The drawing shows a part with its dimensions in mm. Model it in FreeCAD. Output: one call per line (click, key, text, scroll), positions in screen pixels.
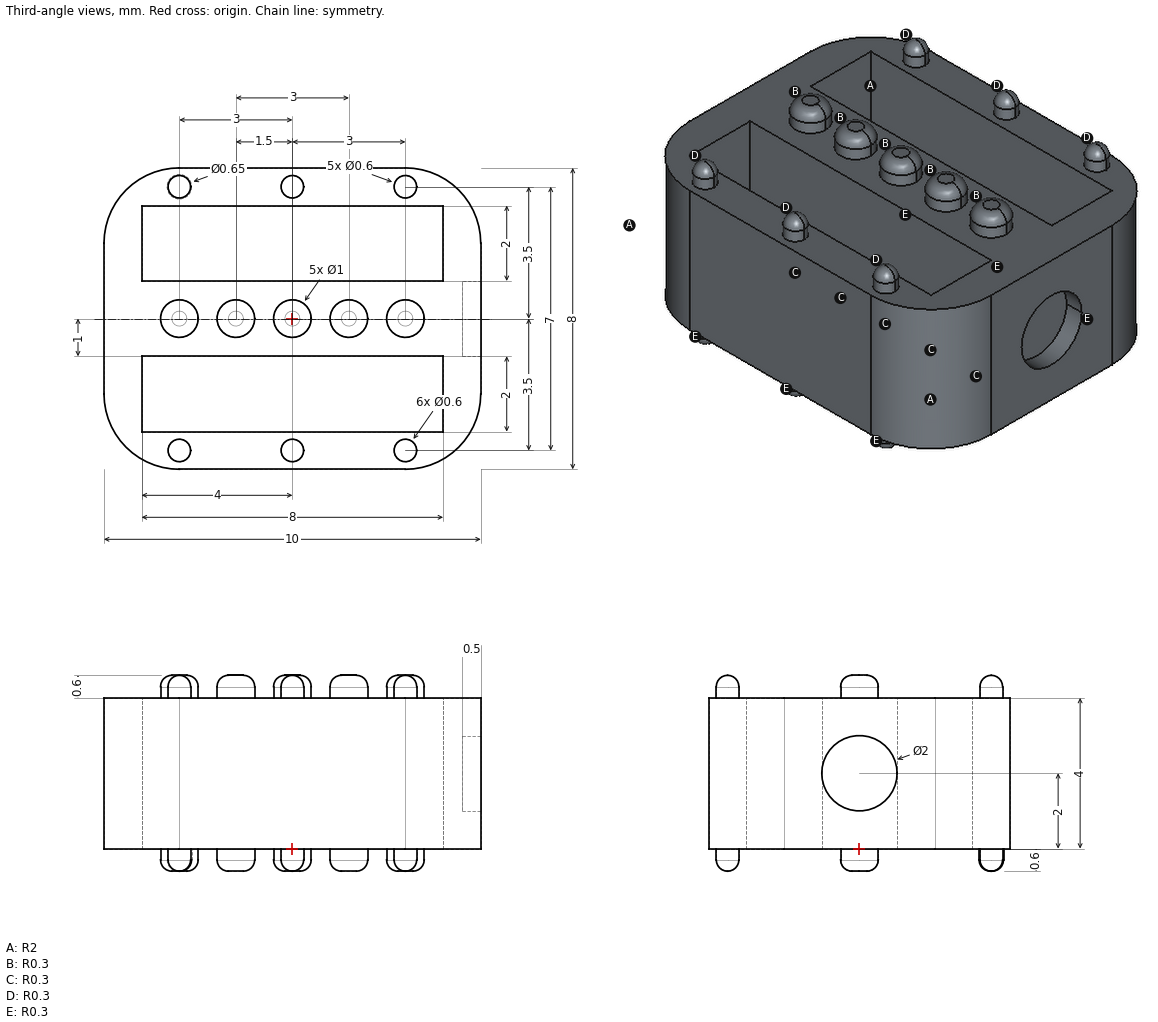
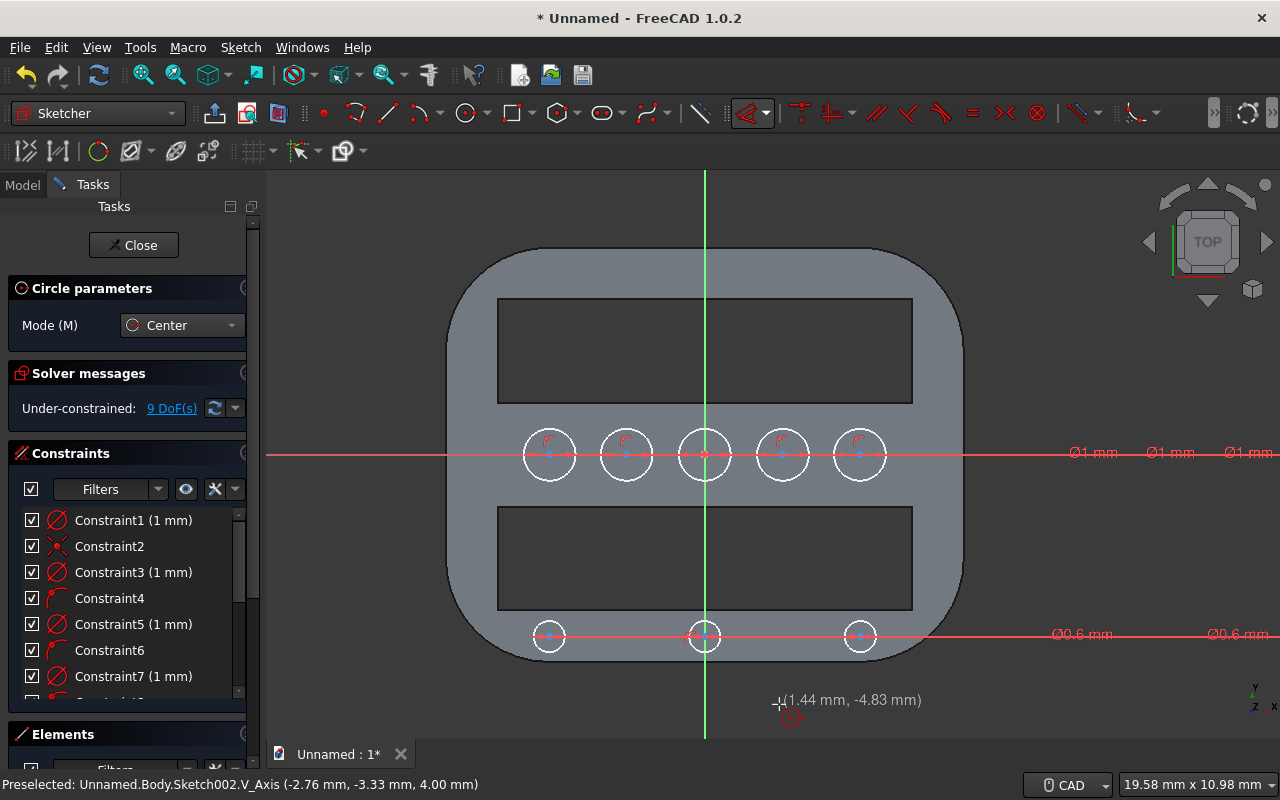
scroll(860, 274, up, 2)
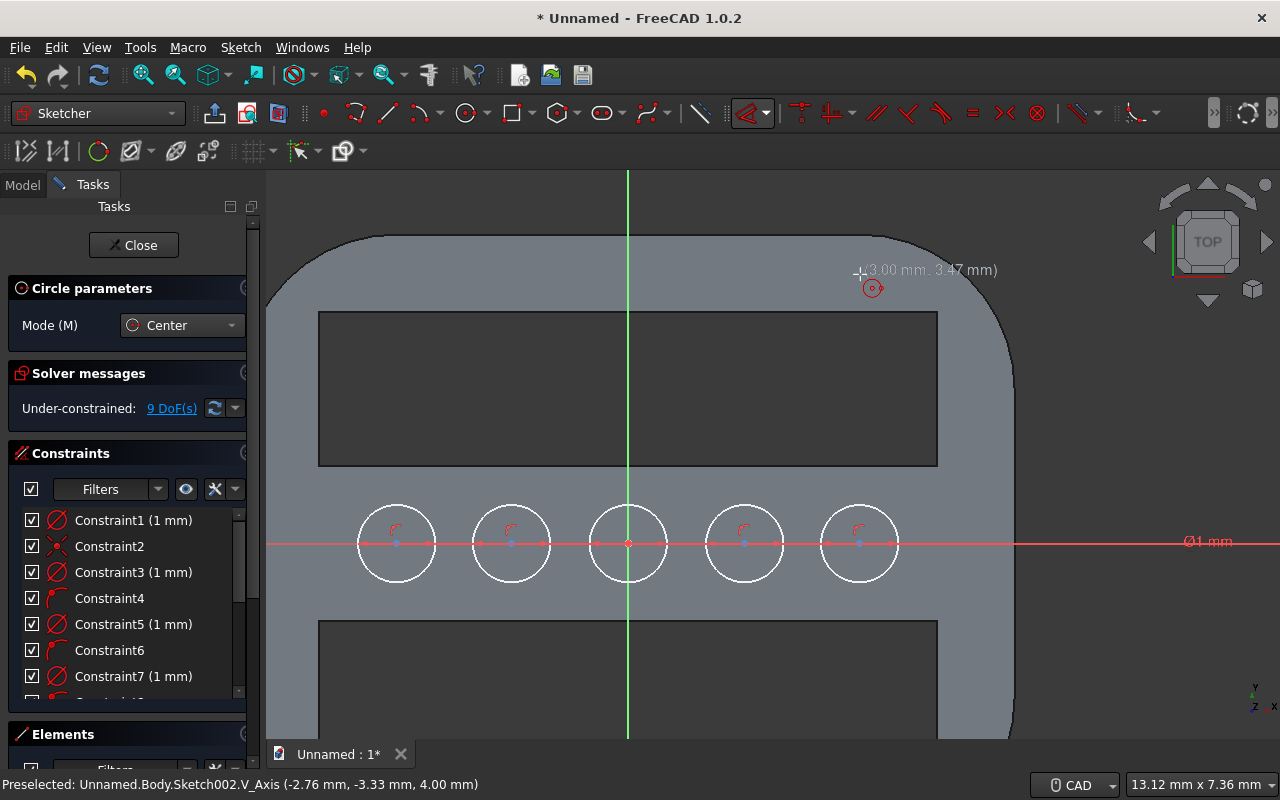
click(860, 273)
move(876, 257)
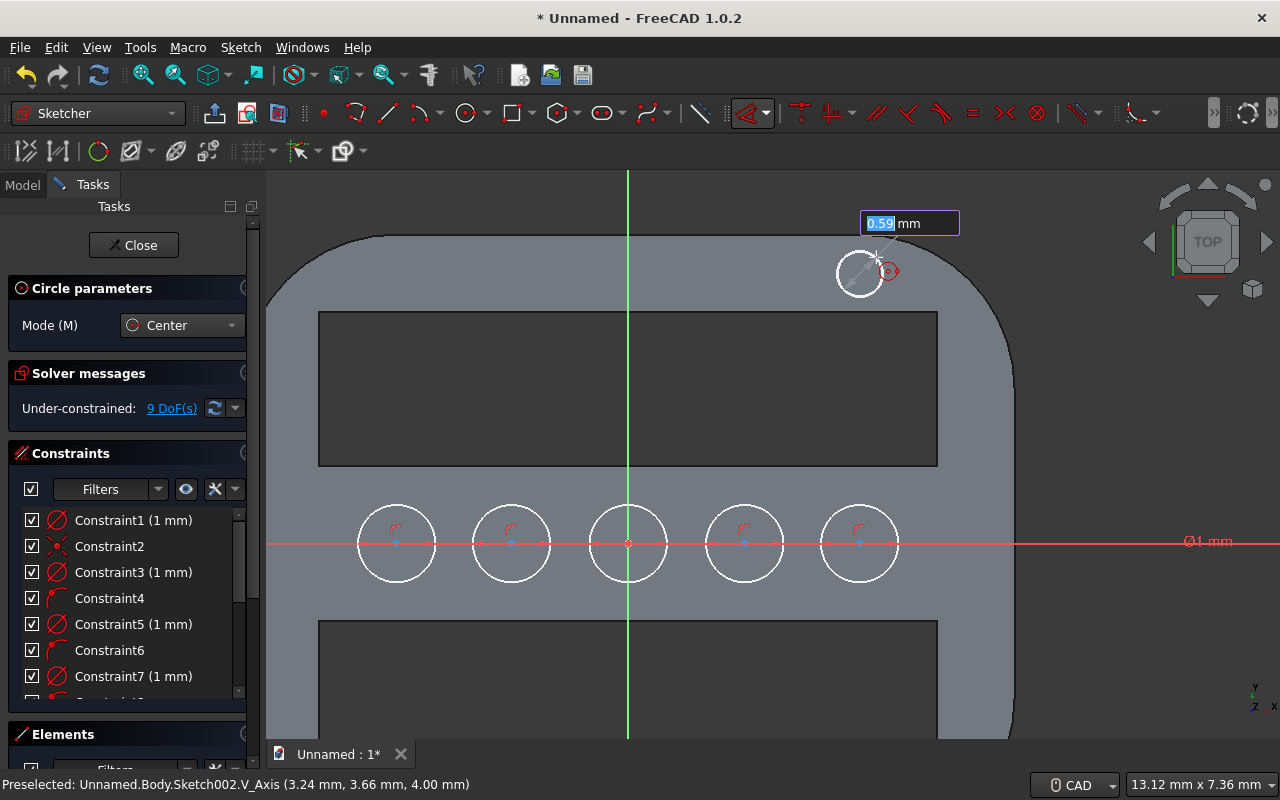
text(0.6)
key(Return)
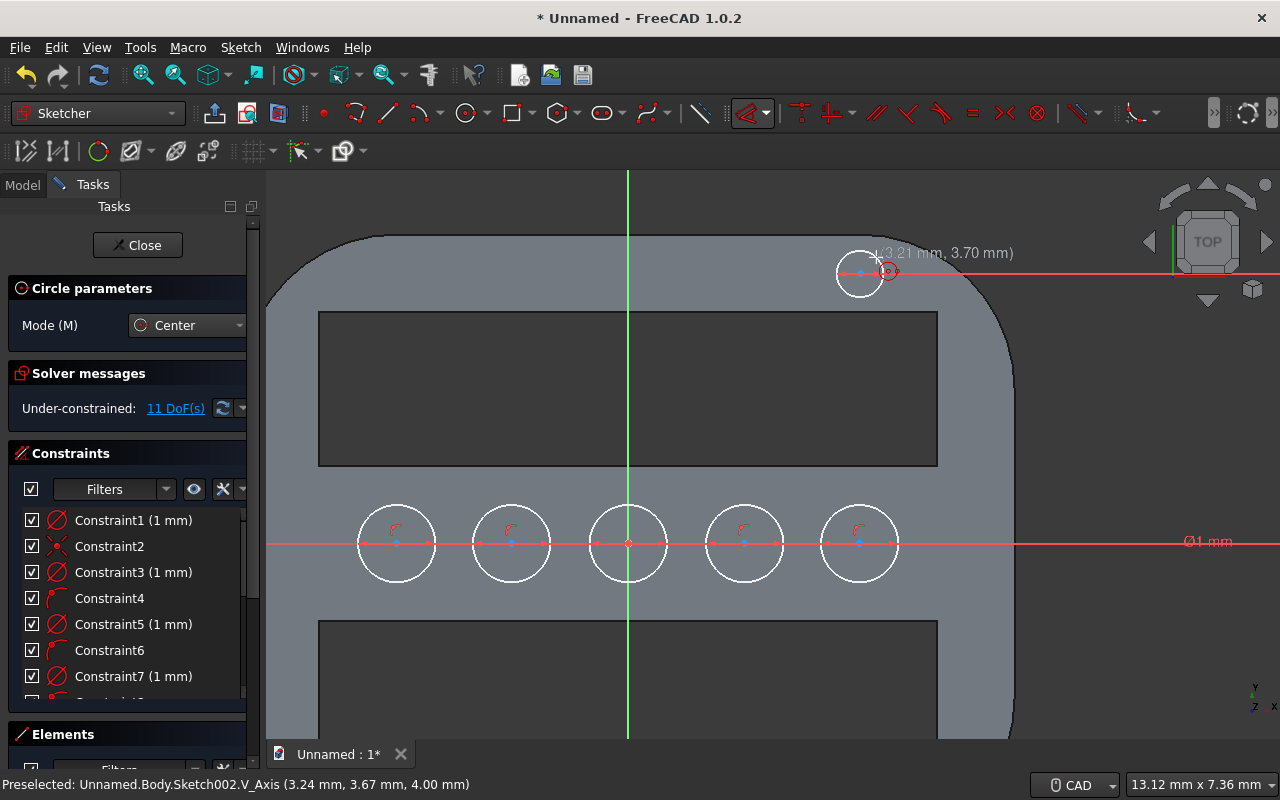
click(628, 273)
move(645, 257)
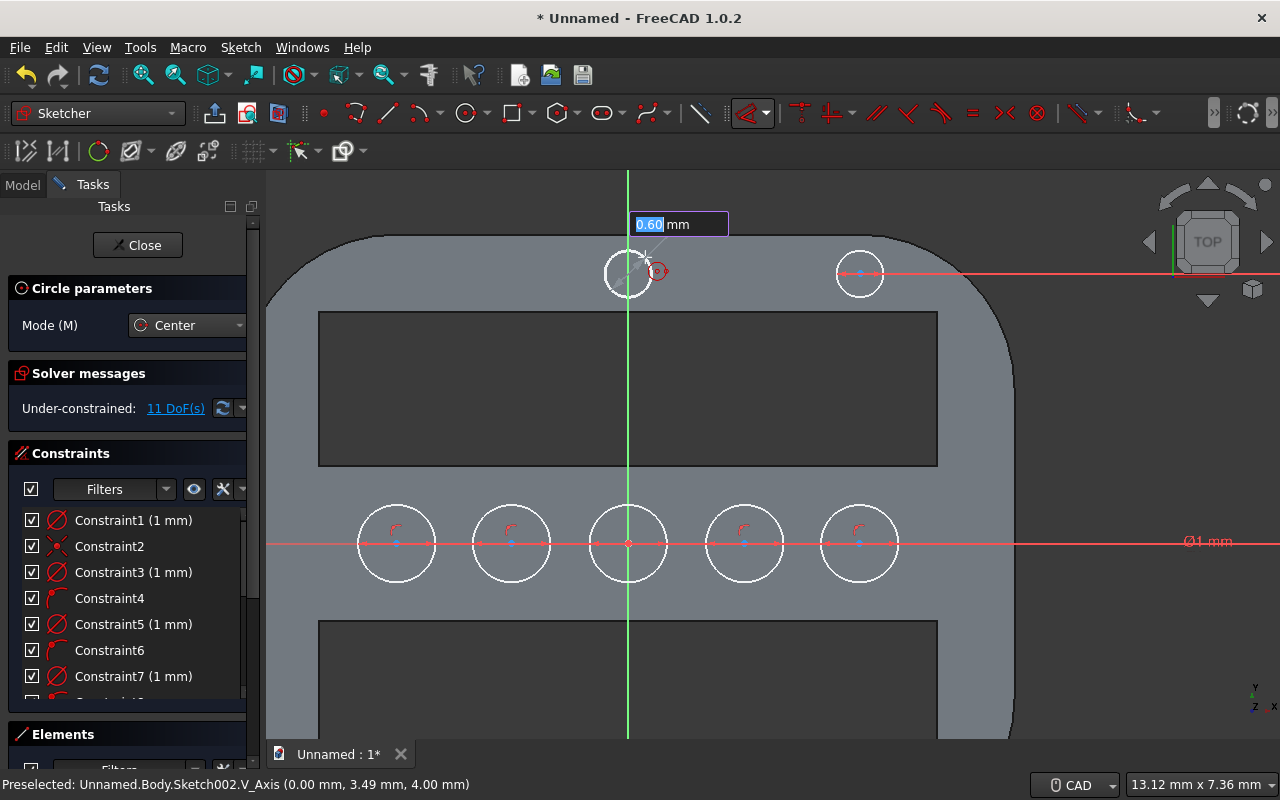
text(0.6)
key(Return)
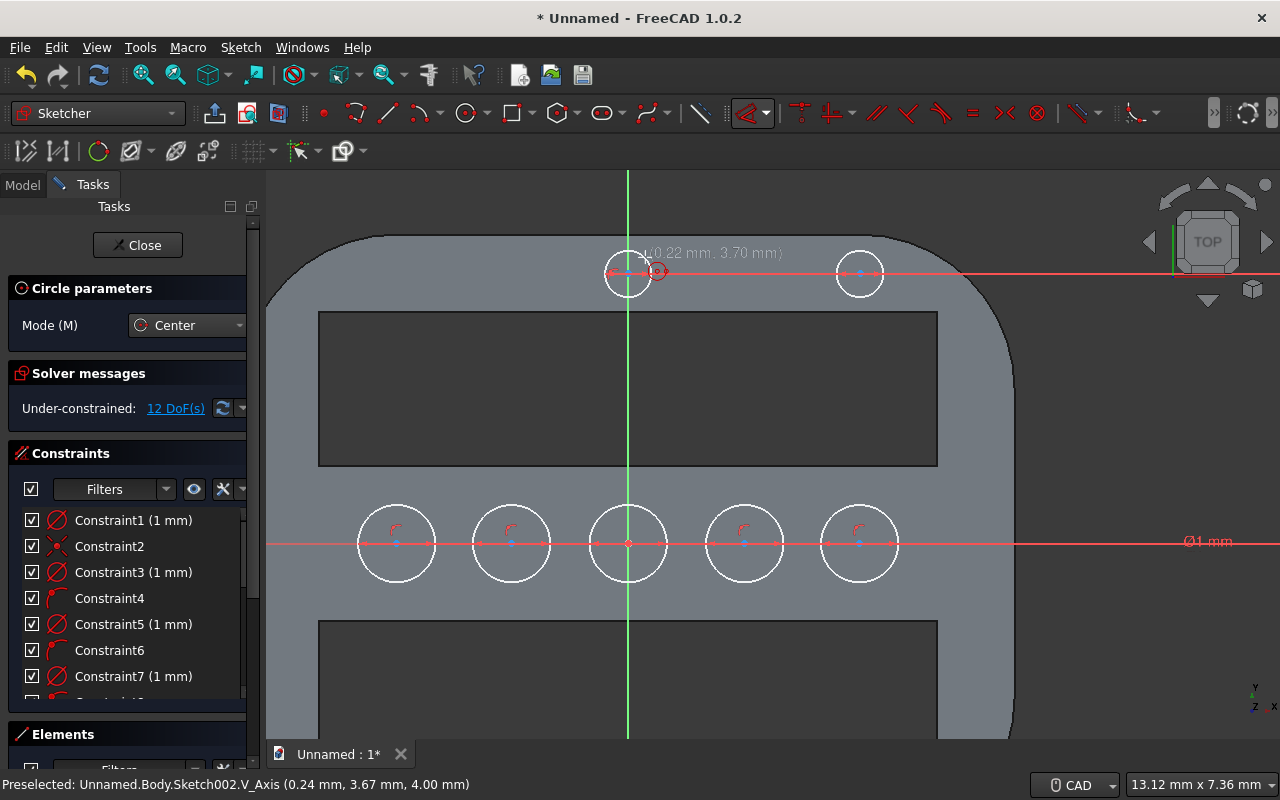
click(396, 273)
move(413, 257)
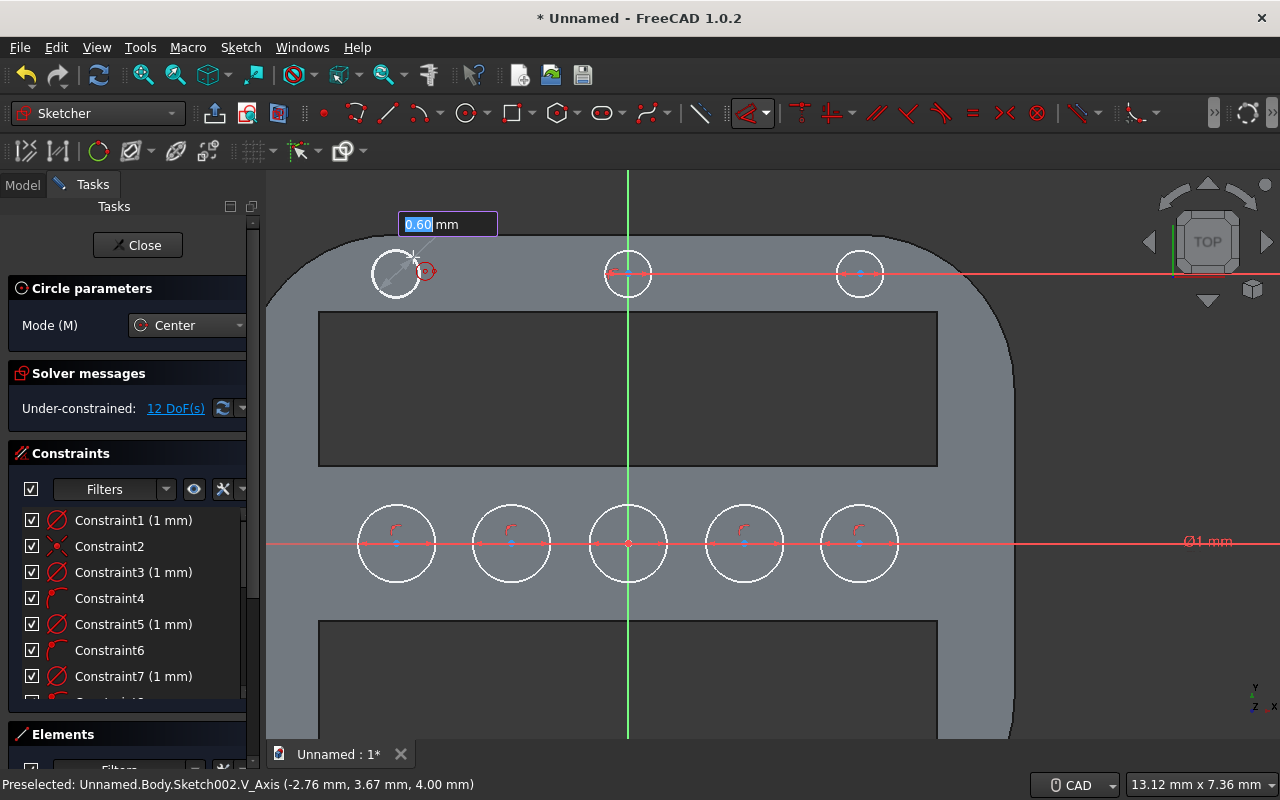
text(0.6)
key(Return)
key(Escape)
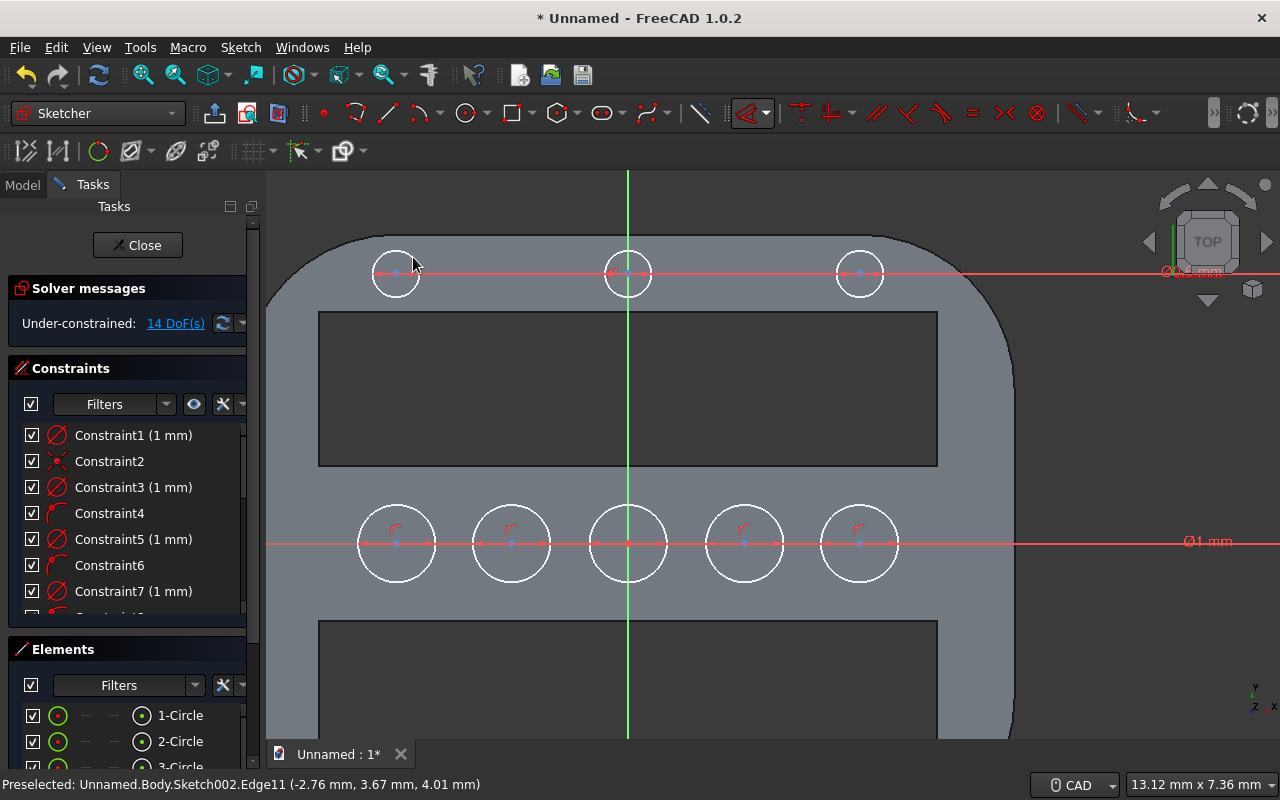
click(860, 544)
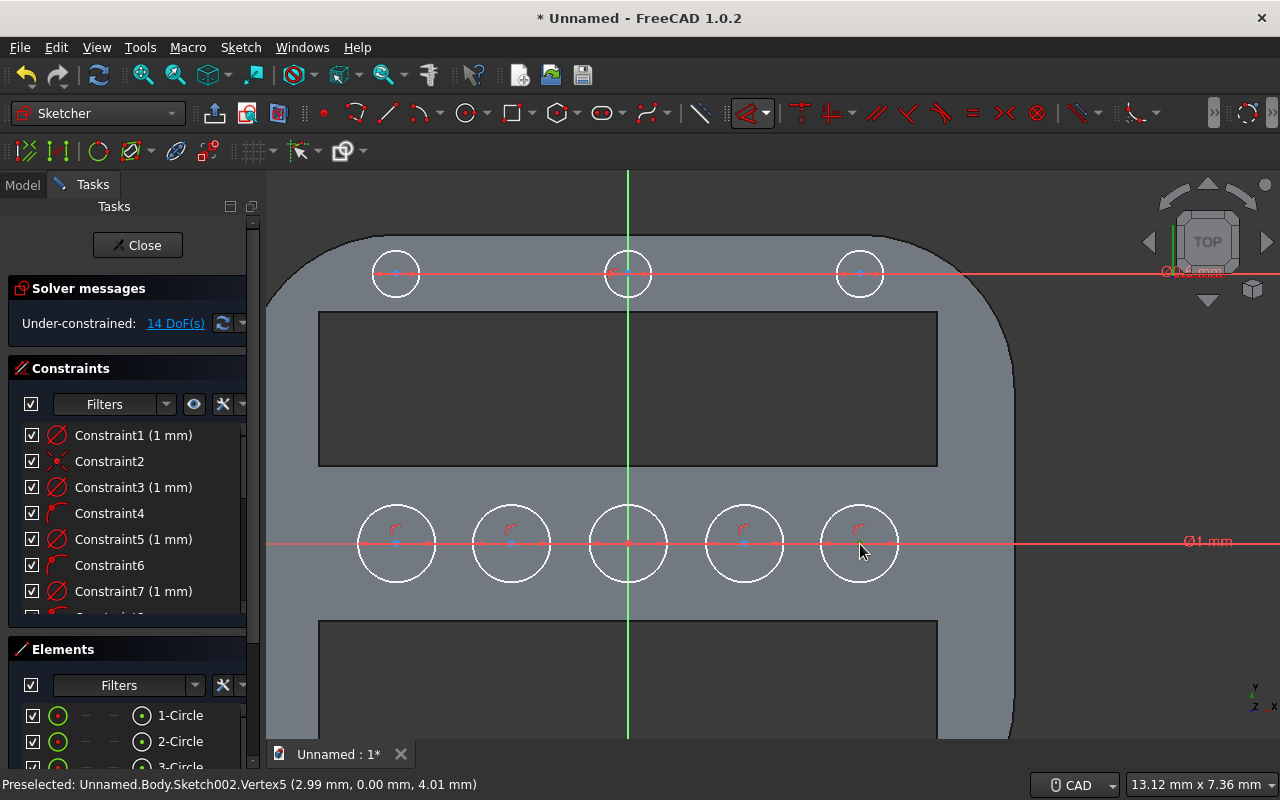
scroll(860, 273, down, 2)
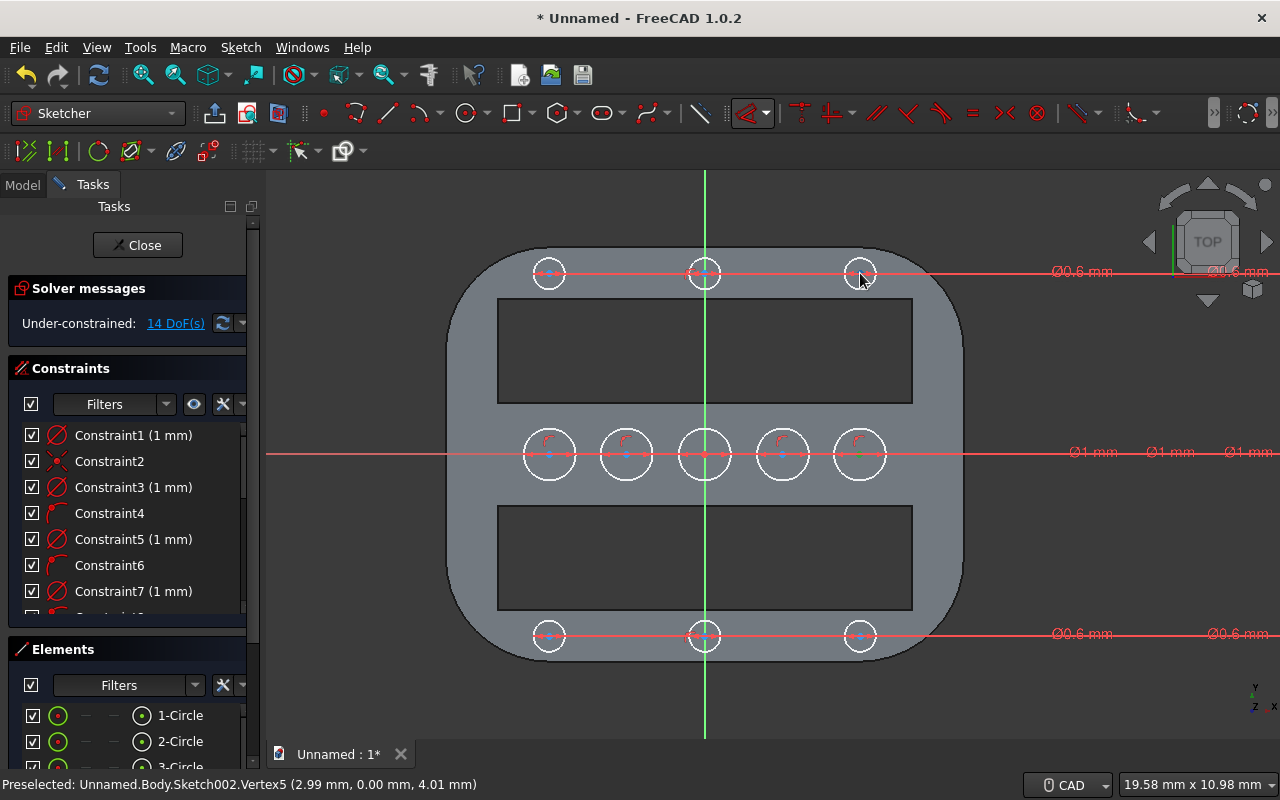
click(860, 636)